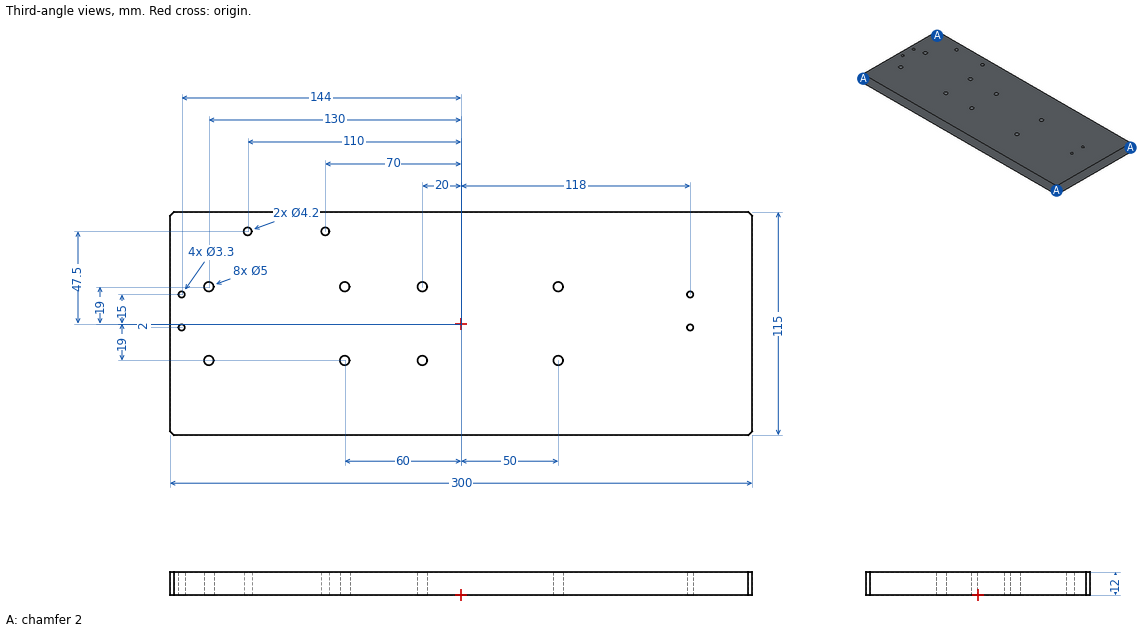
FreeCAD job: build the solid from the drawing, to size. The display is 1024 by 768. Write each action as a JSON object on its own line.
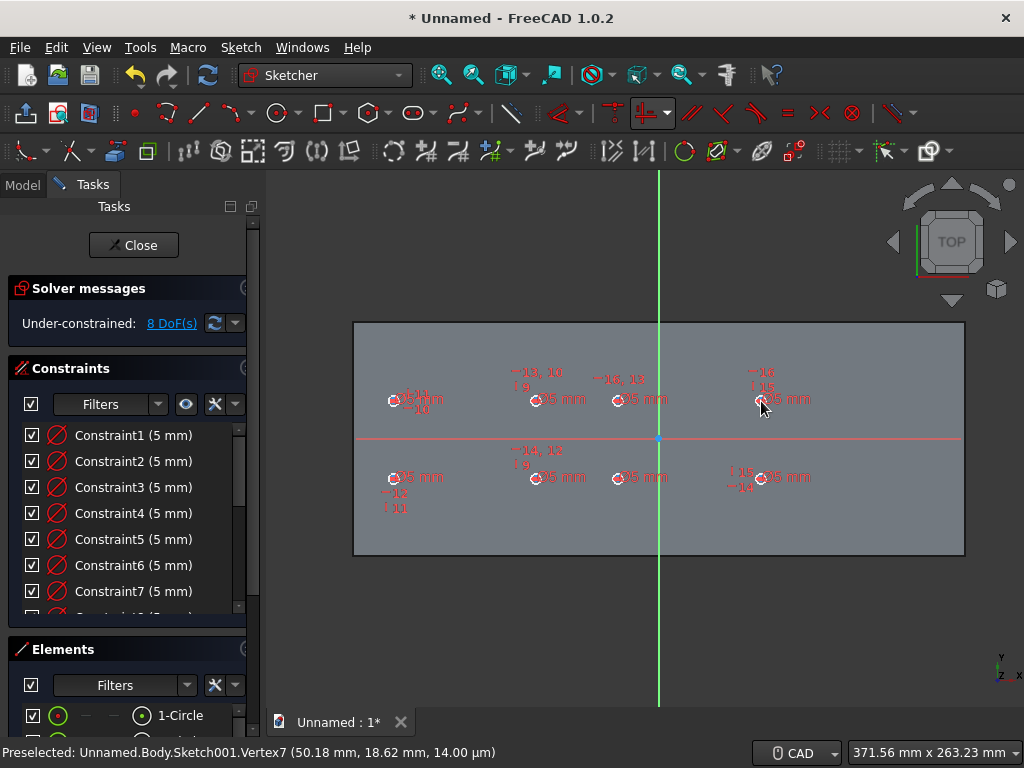
{"action": "left_click", "coordinate": [618, 401]}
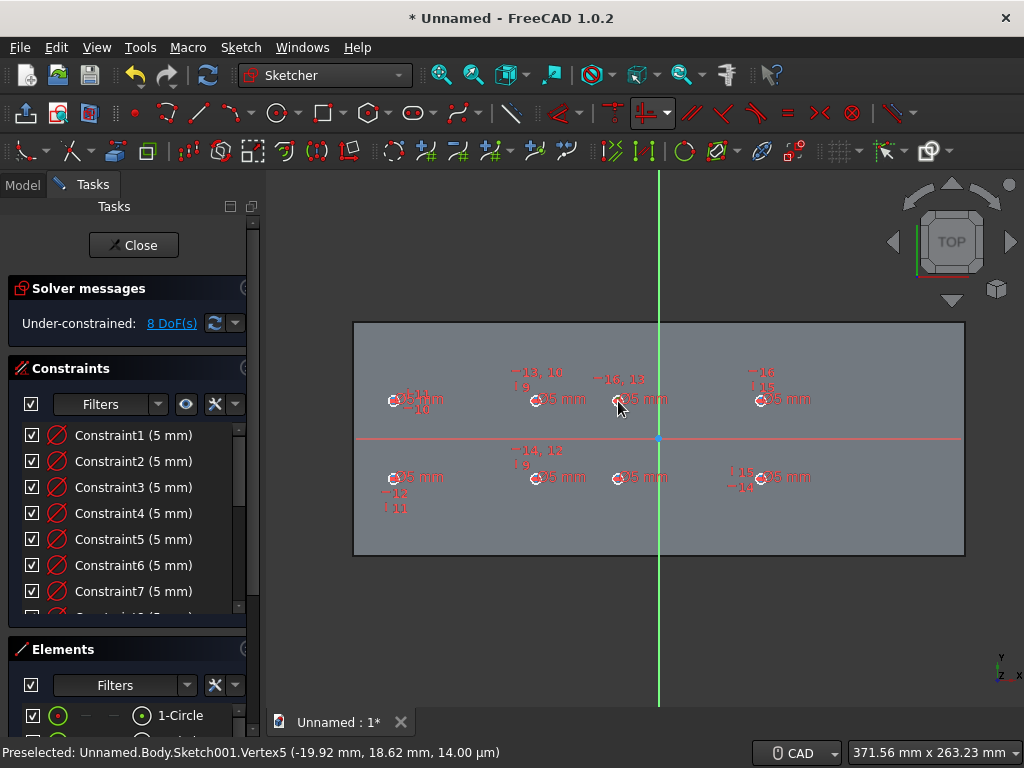
{"action": "left_click", "coordinate": [618, 479]}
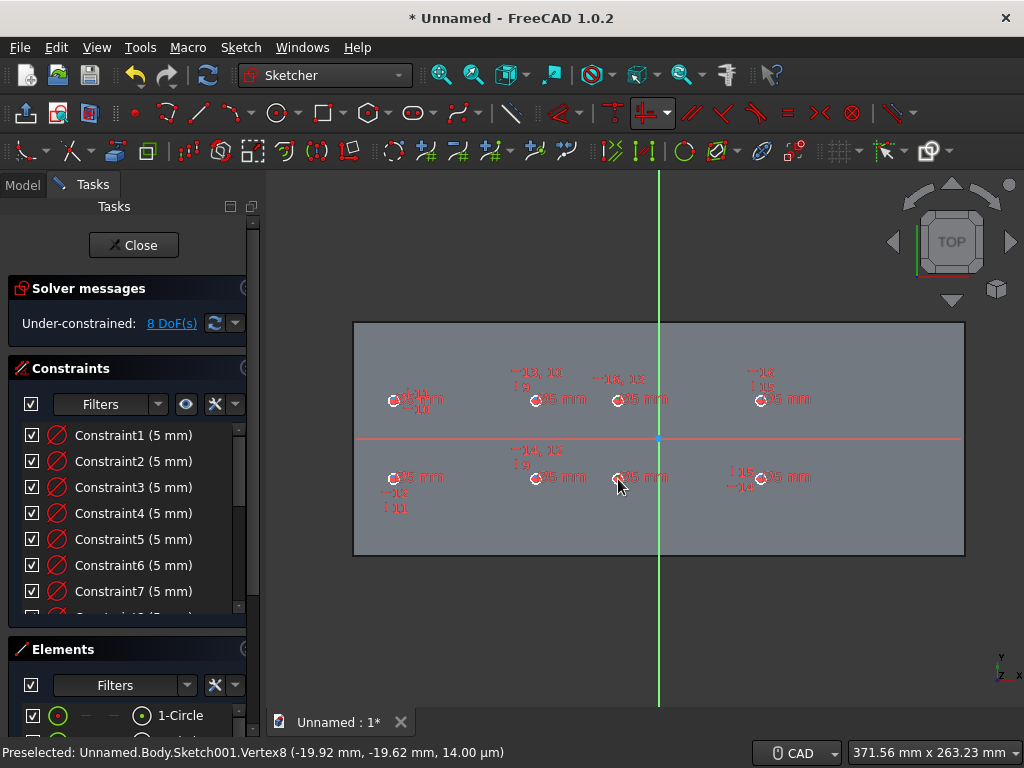
{"action": "left_click", "coordinate": [670, 114]}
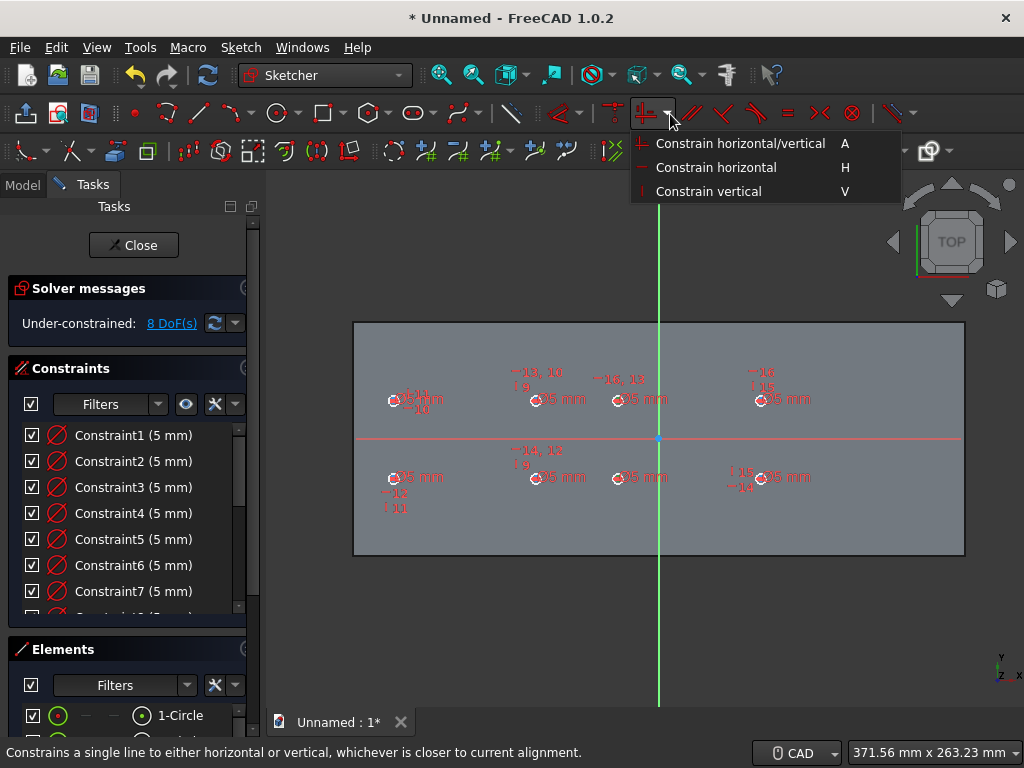
{"action": "left_click", "coordinate": [766, 191]}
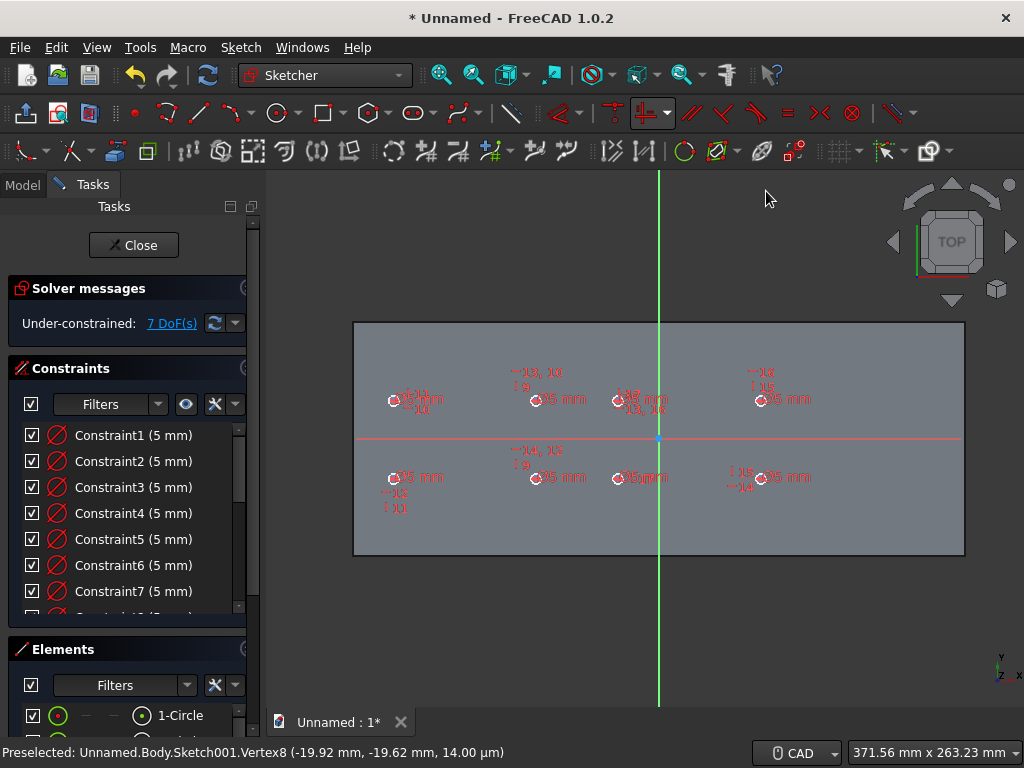
{"action": "left_click", "coordinate": [536, 479]}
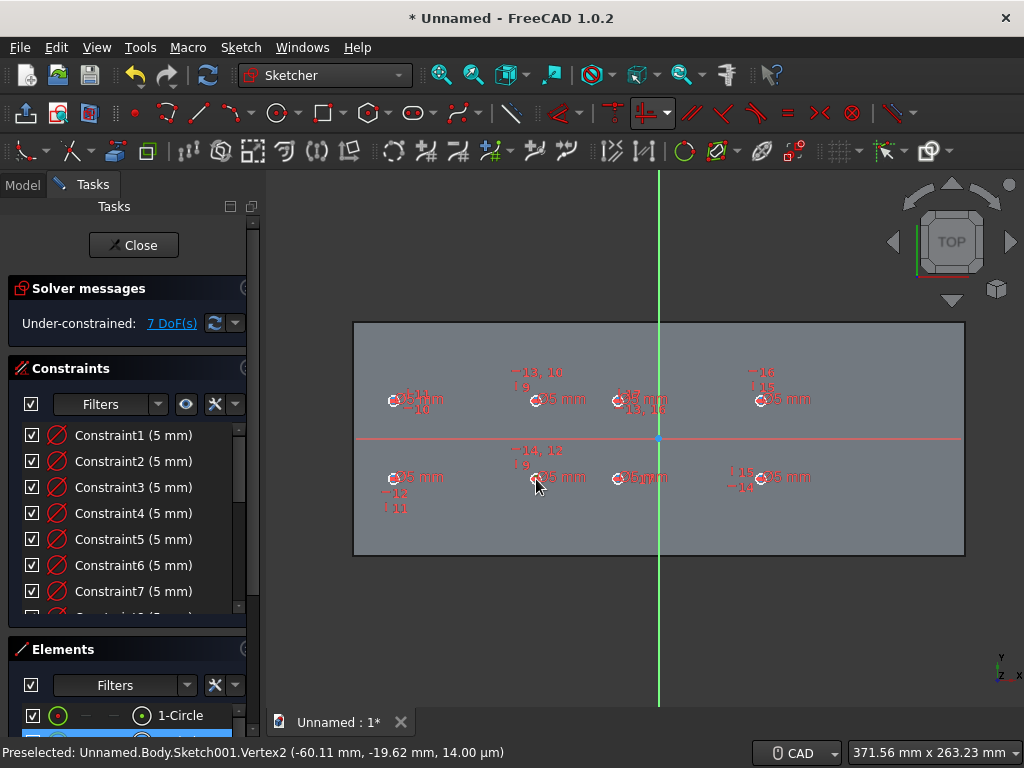
{"action": "left_click", "coordinate": [618, 479]}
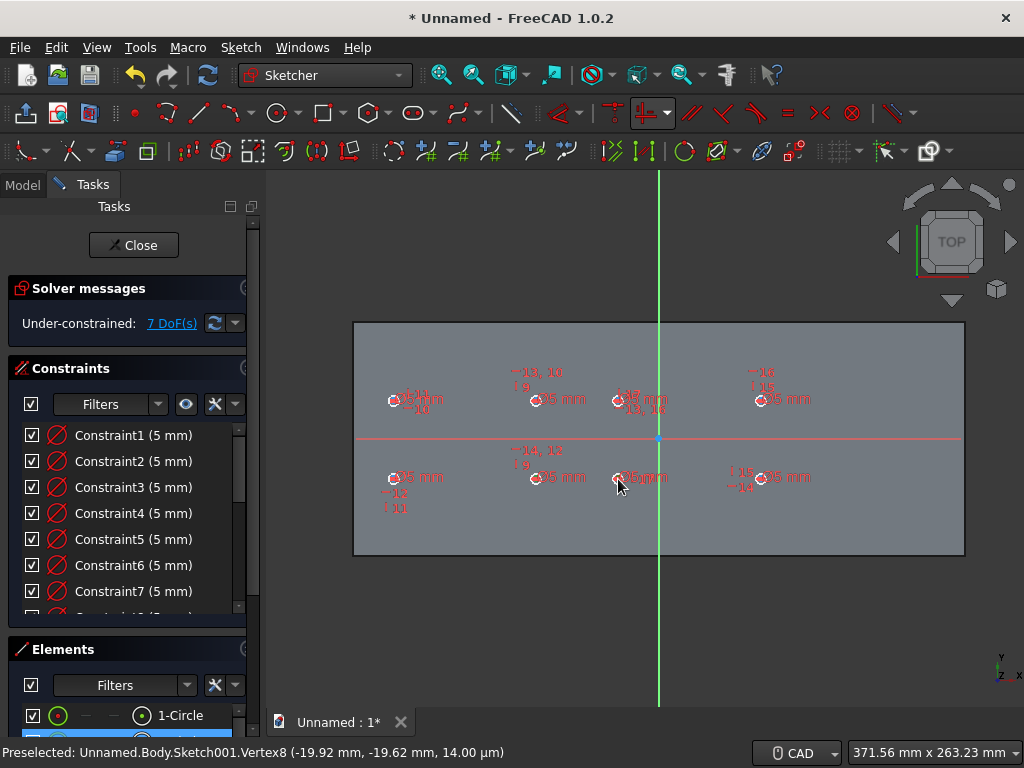
{"action": "left_click", "coordinate": [670, 114]}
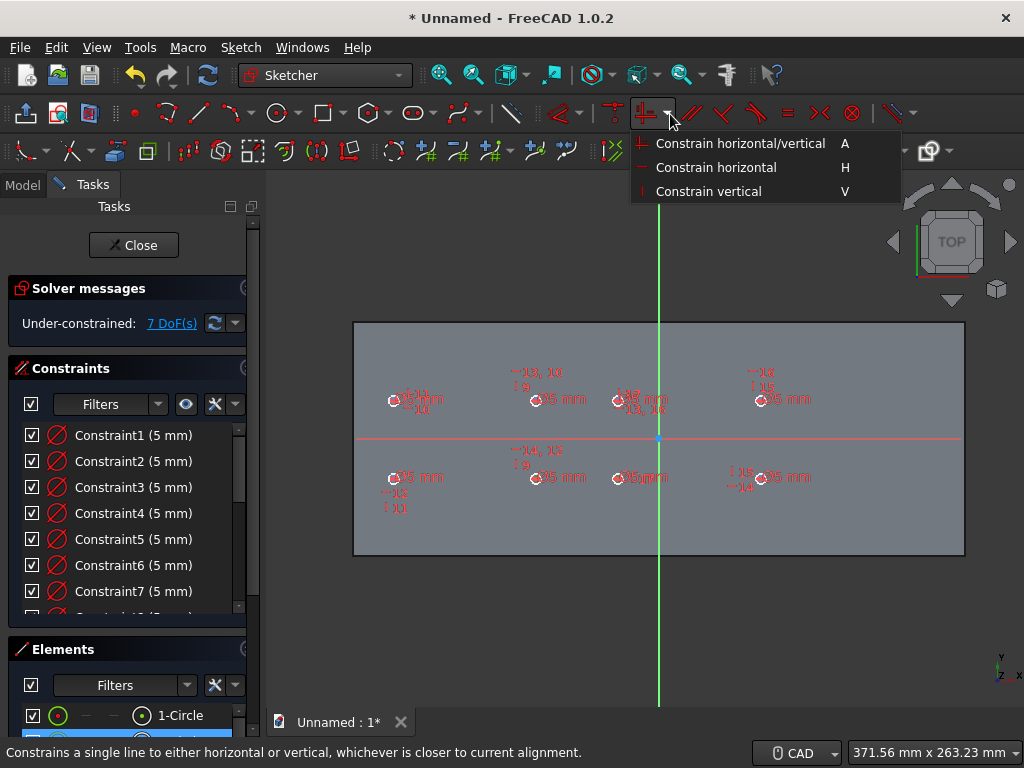
{"action": "left_click", "coordinate": [766, 167]}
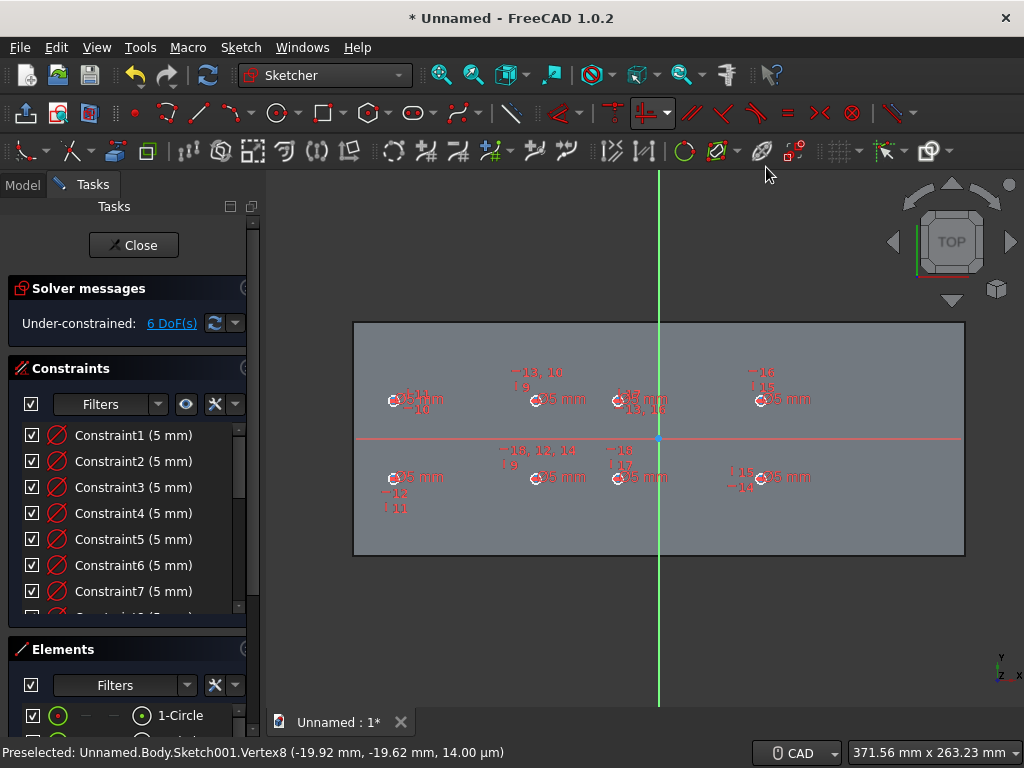
{"action": "left_click", "coordinate": [558, 114]}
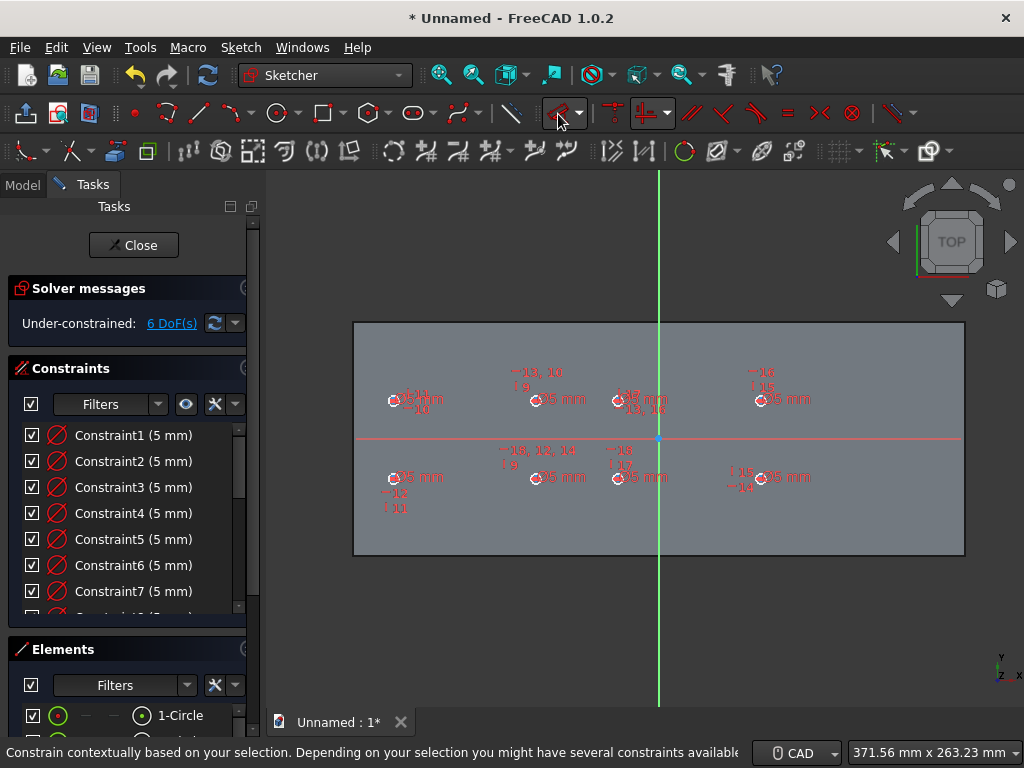
{"action": "left_click", "coordinate": [394, 401]}
{"action": "left_click", "coordinate": [360, 420]}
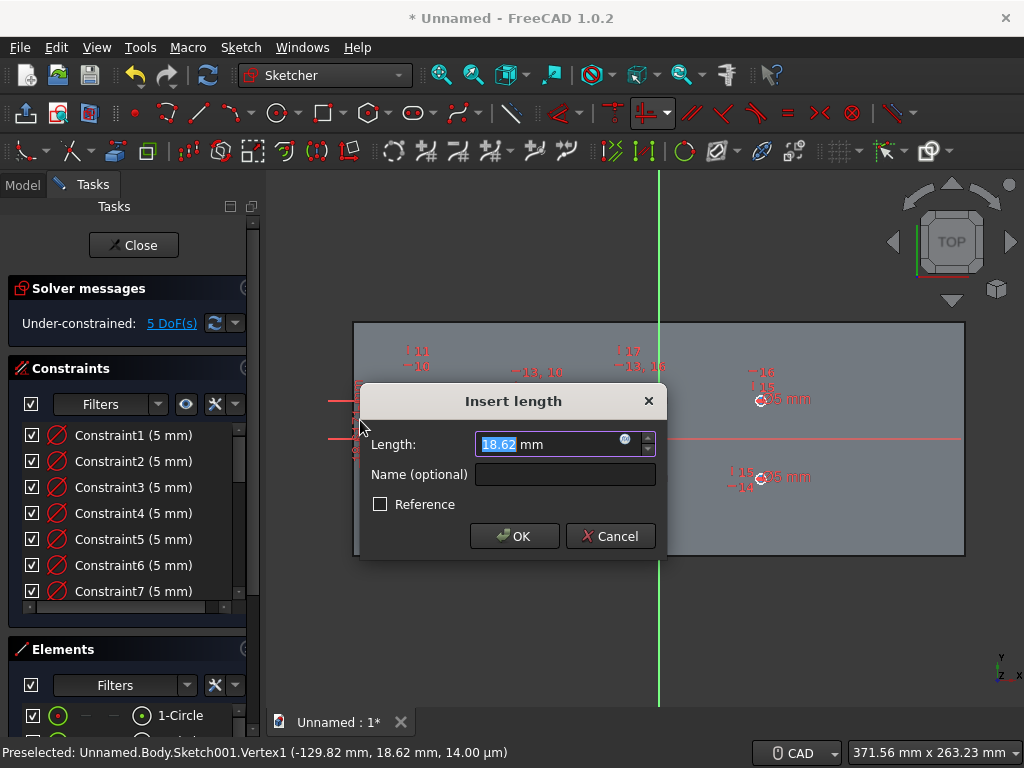
{"action": "type", "text": "19"}
{"action": "key", "text": "Return"}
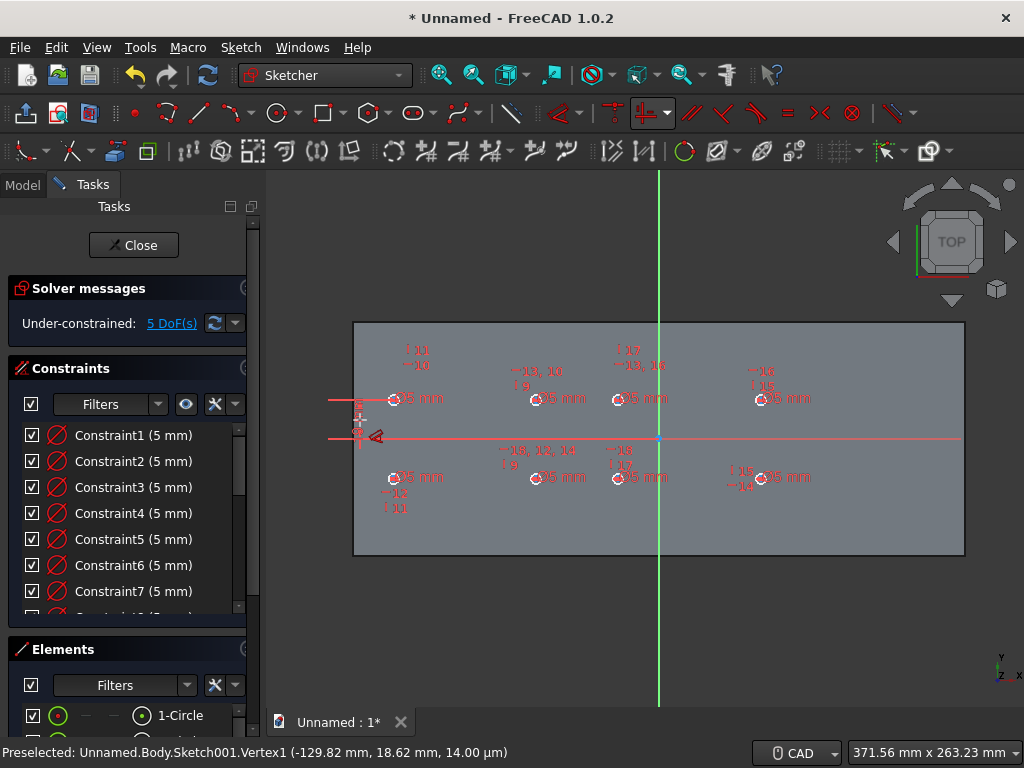
{"action": "left_click", "coordinate": [536, 479]}
{"action": "left_click", "coordinate": [597, 513]}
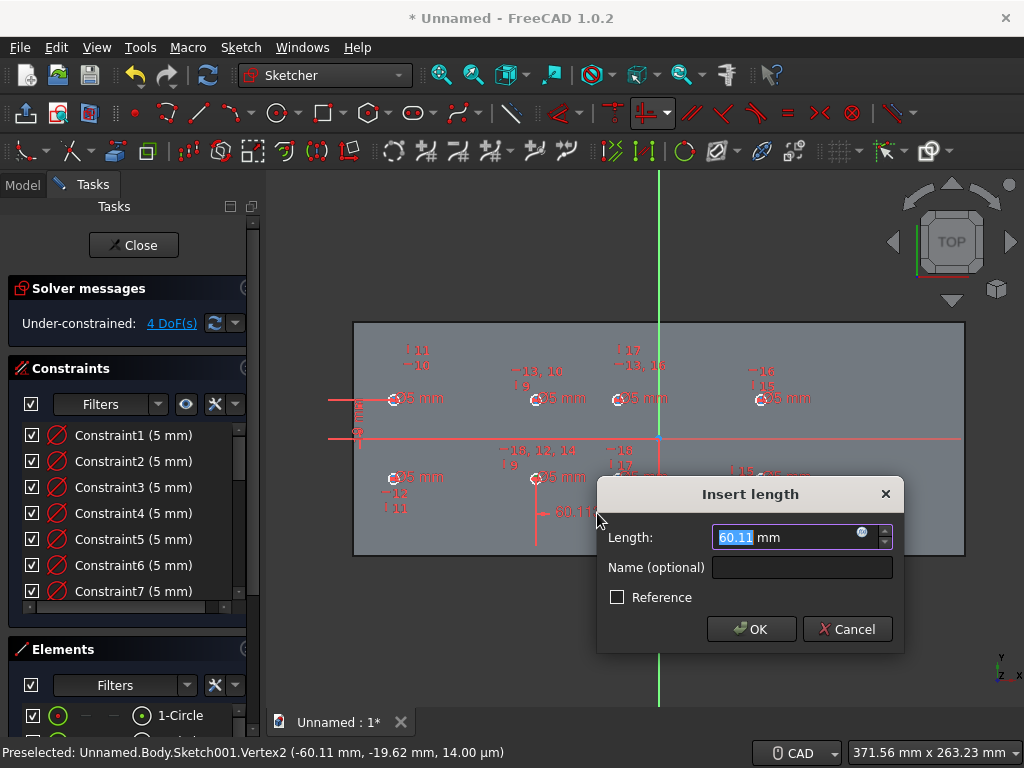
{"action": "type", "text": "60"}
{"action": "key", "text": "Return"}